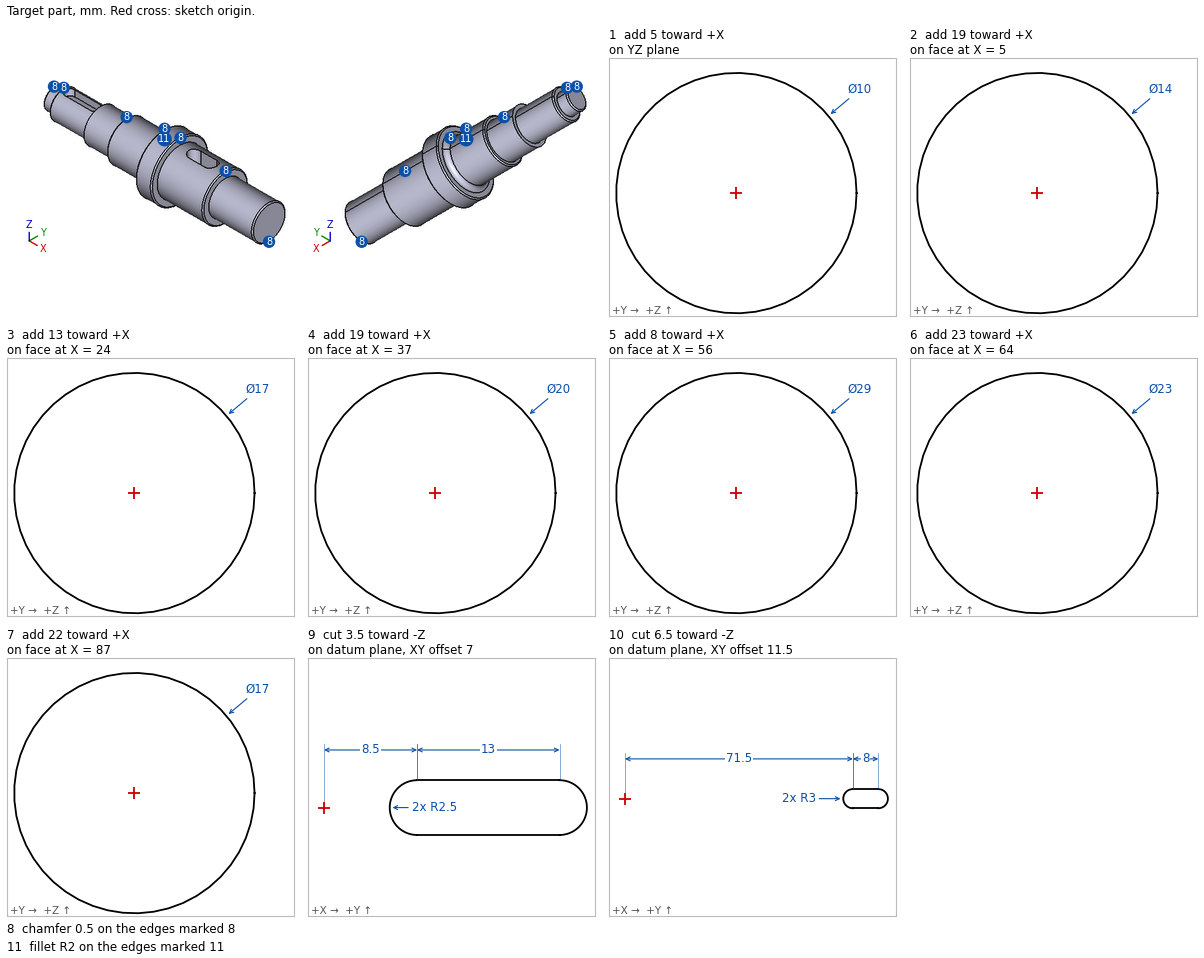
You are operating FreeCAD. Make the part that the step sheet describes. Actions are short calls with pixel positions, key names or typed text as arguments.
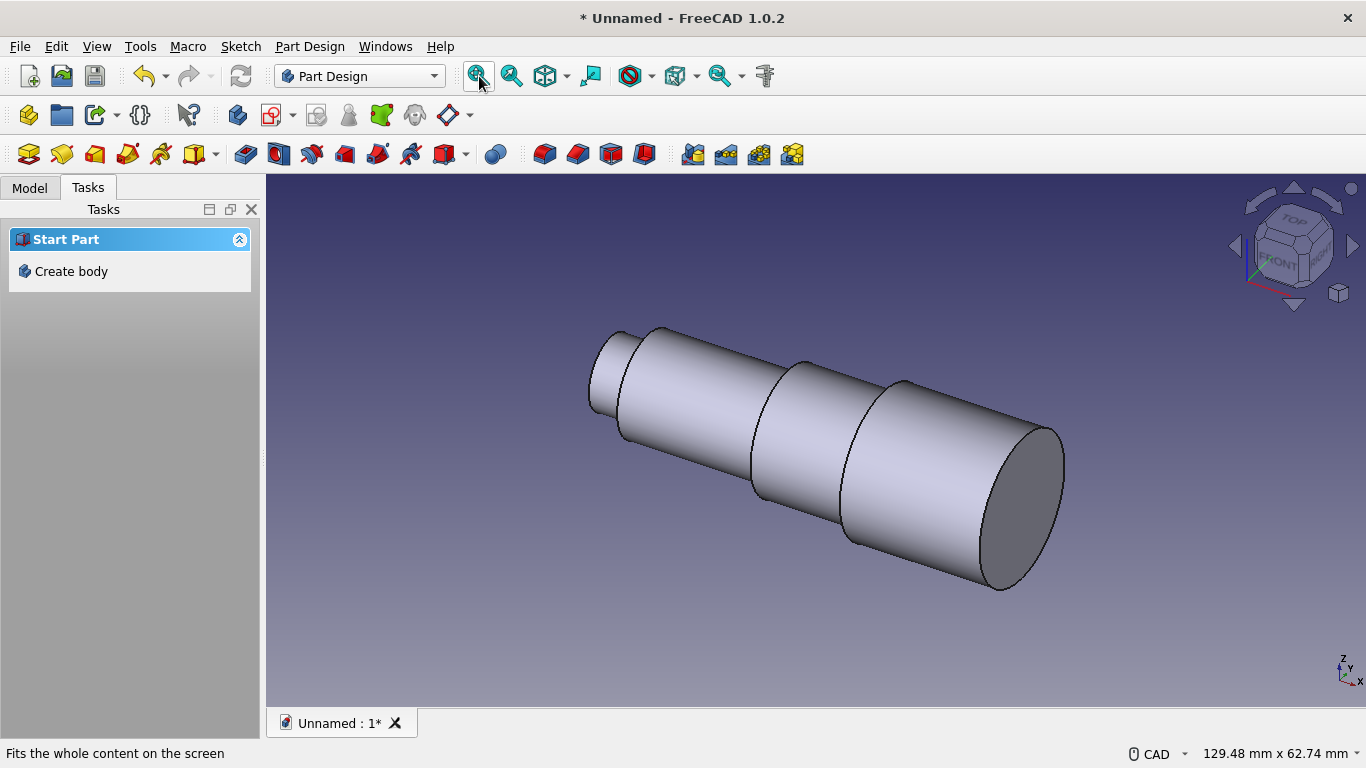
click(1022, 508)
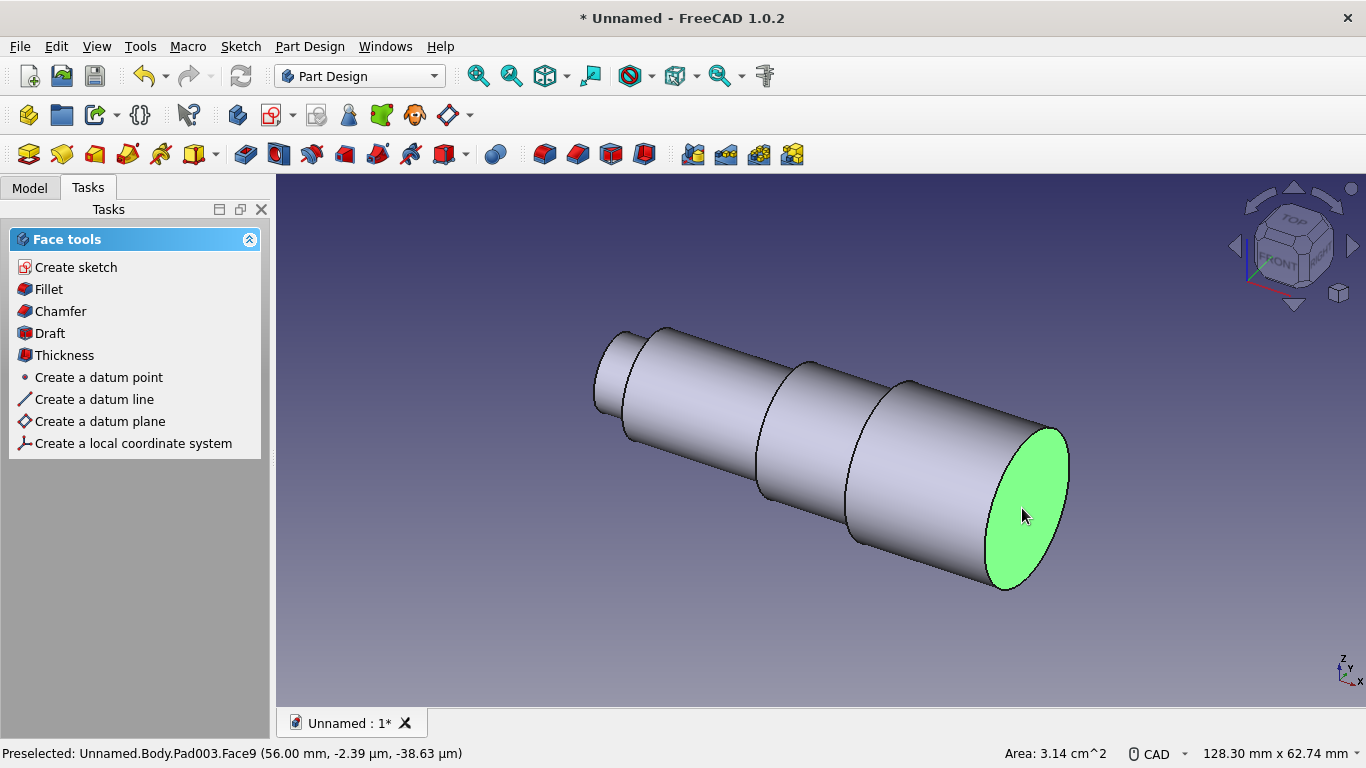
click(270, 116)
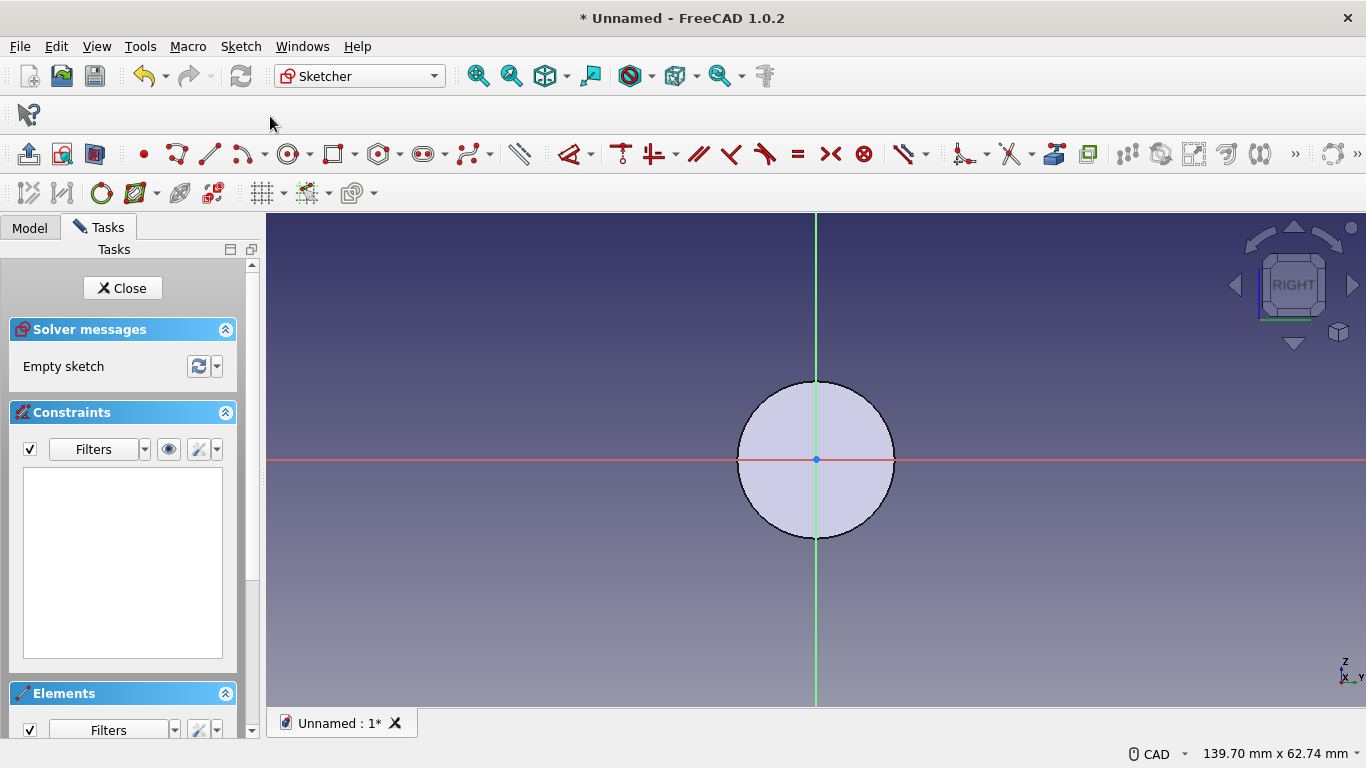
scroll(955, 460, up, 2)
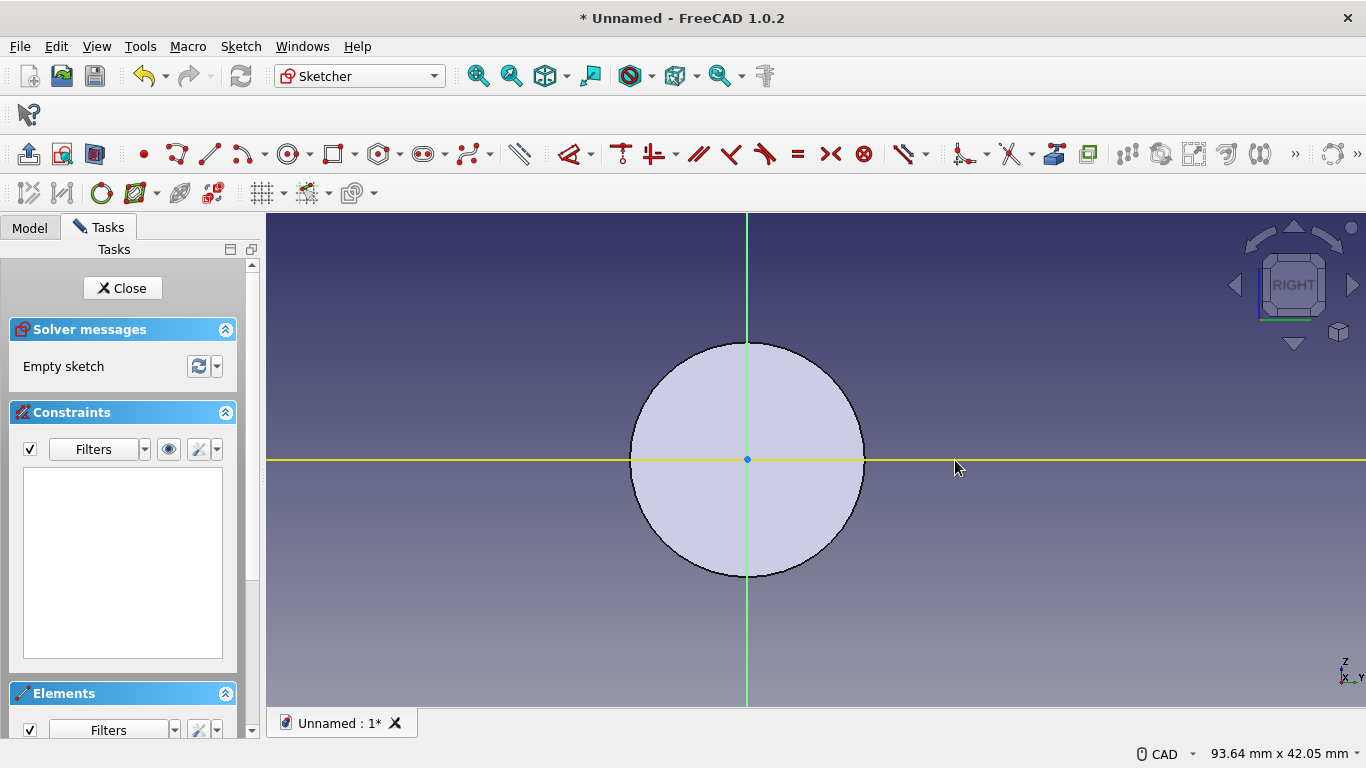
key(g)
key(c)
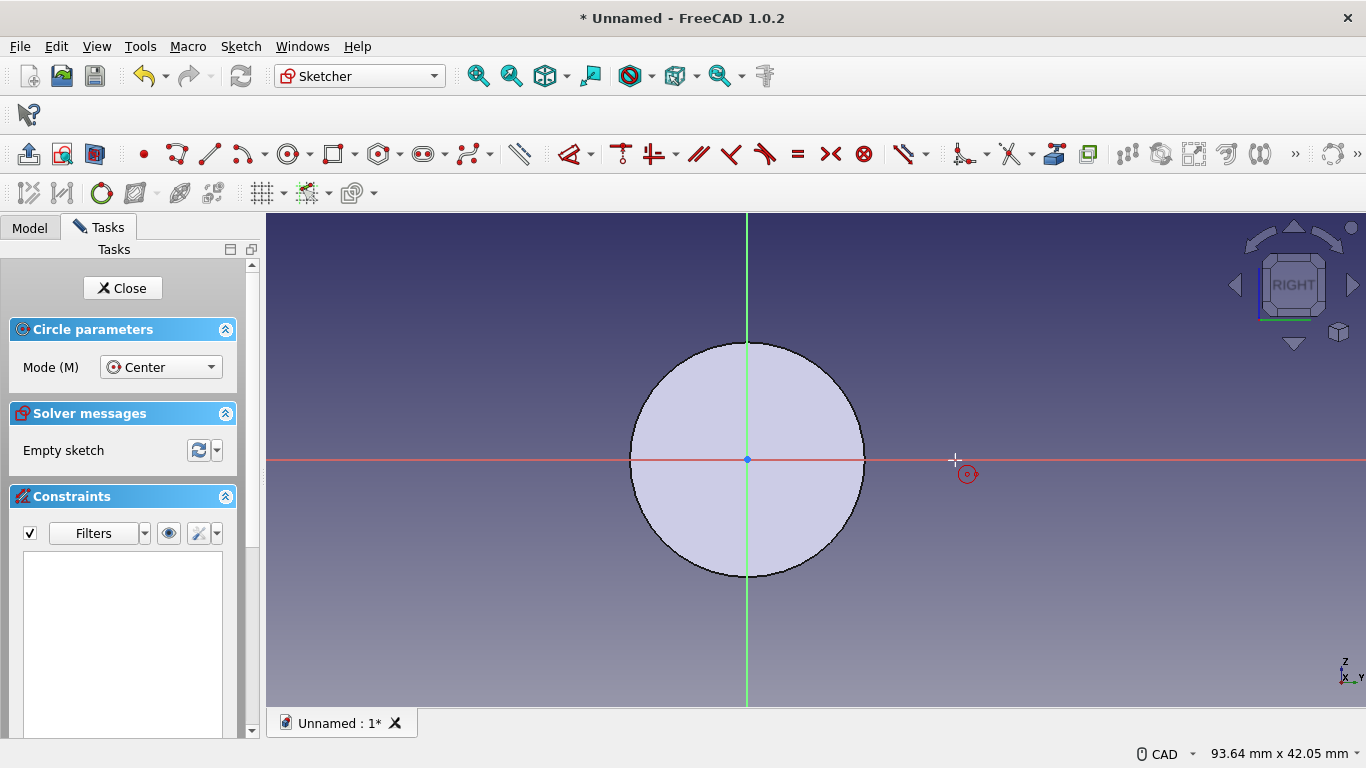
click(747, 460)
move(868, 339)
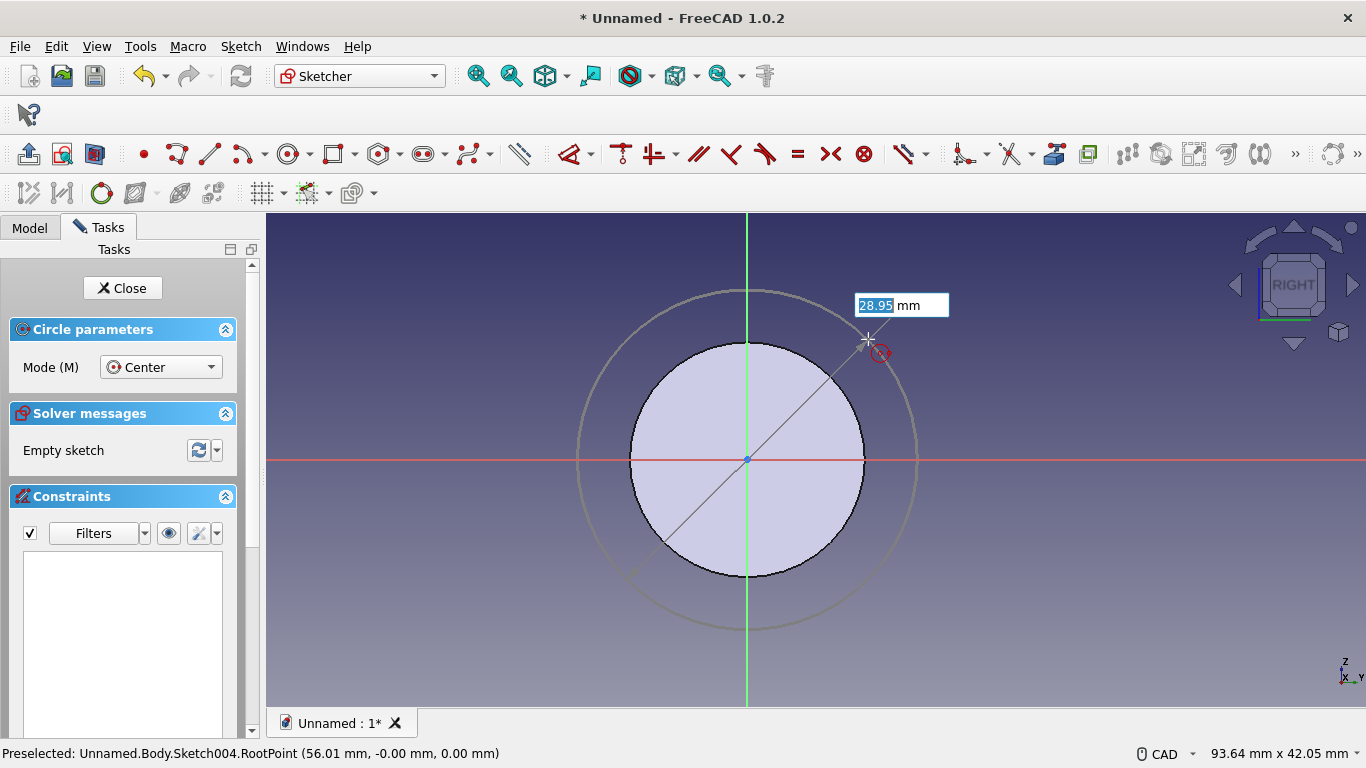
text(29)
key(Return)
key(Escape)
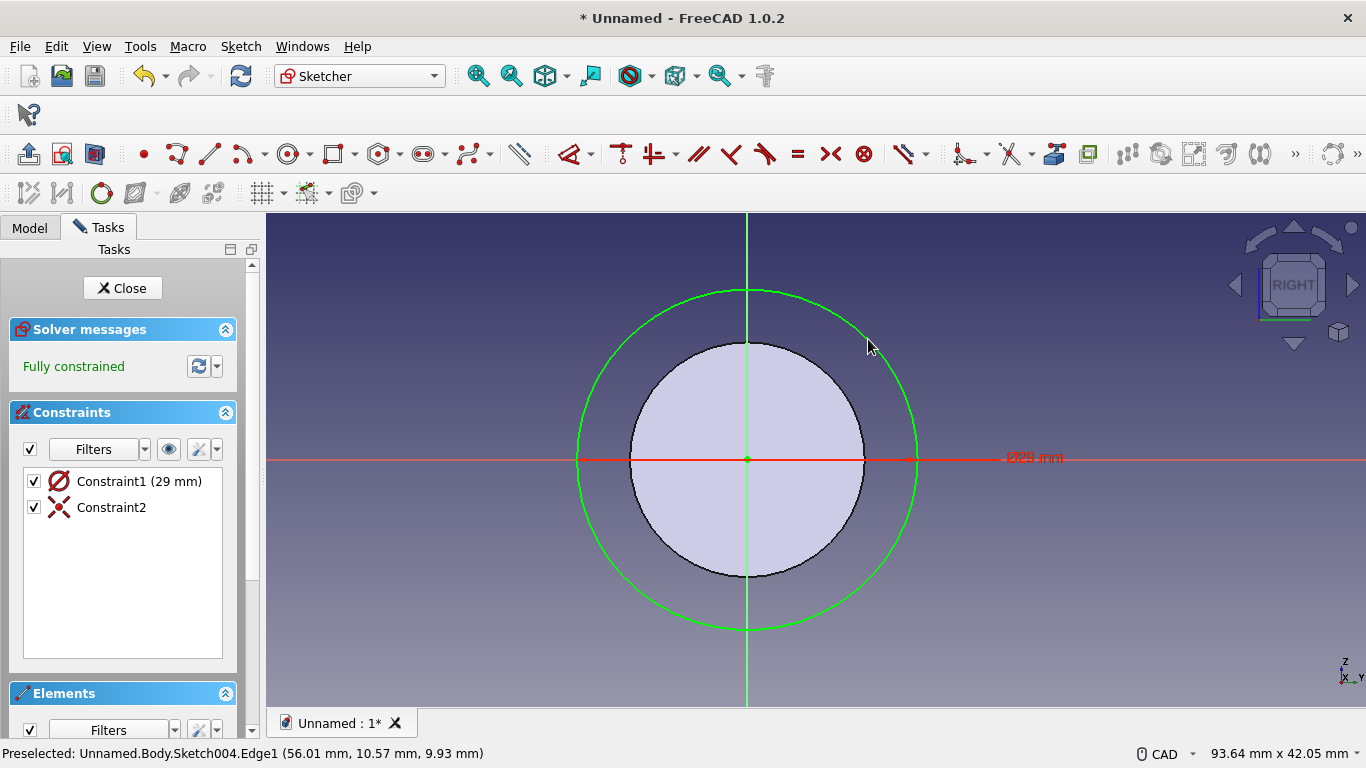
click(123, 288)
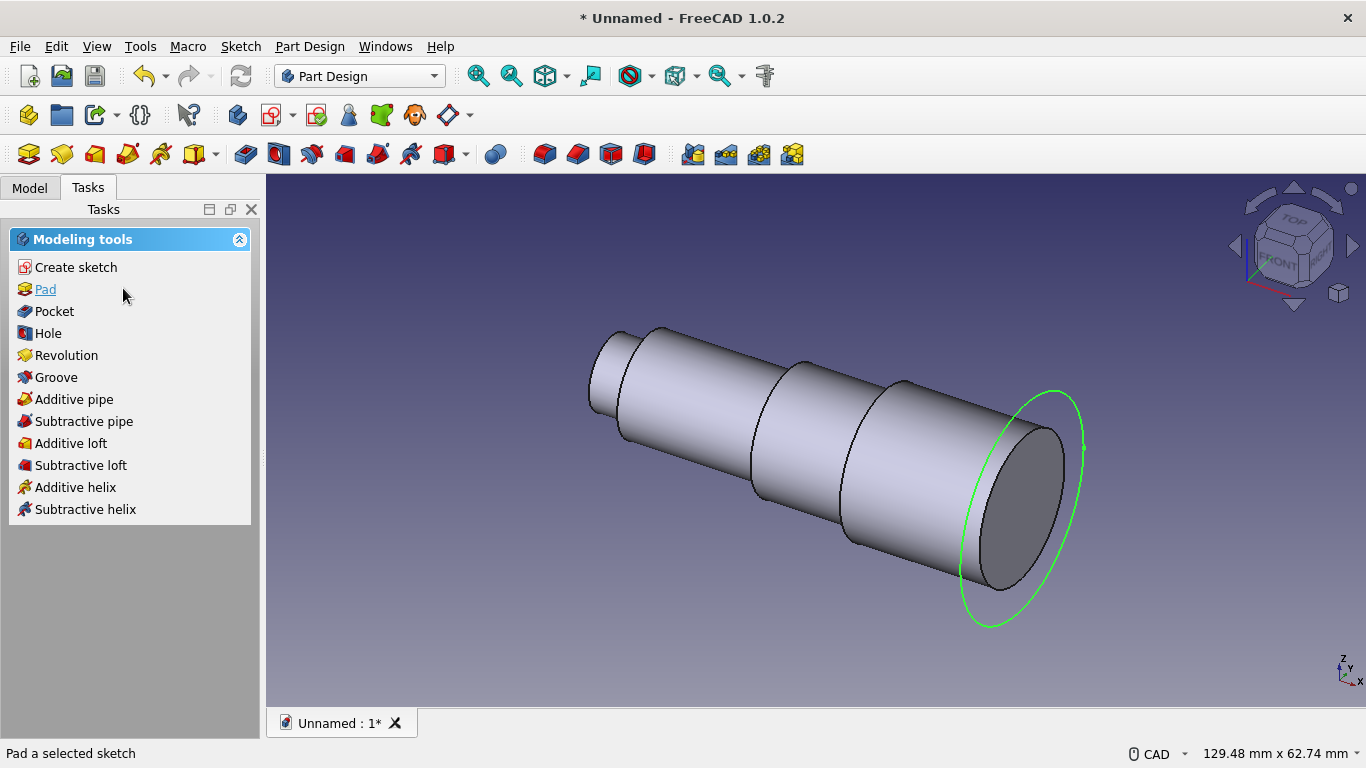
click(29, 154)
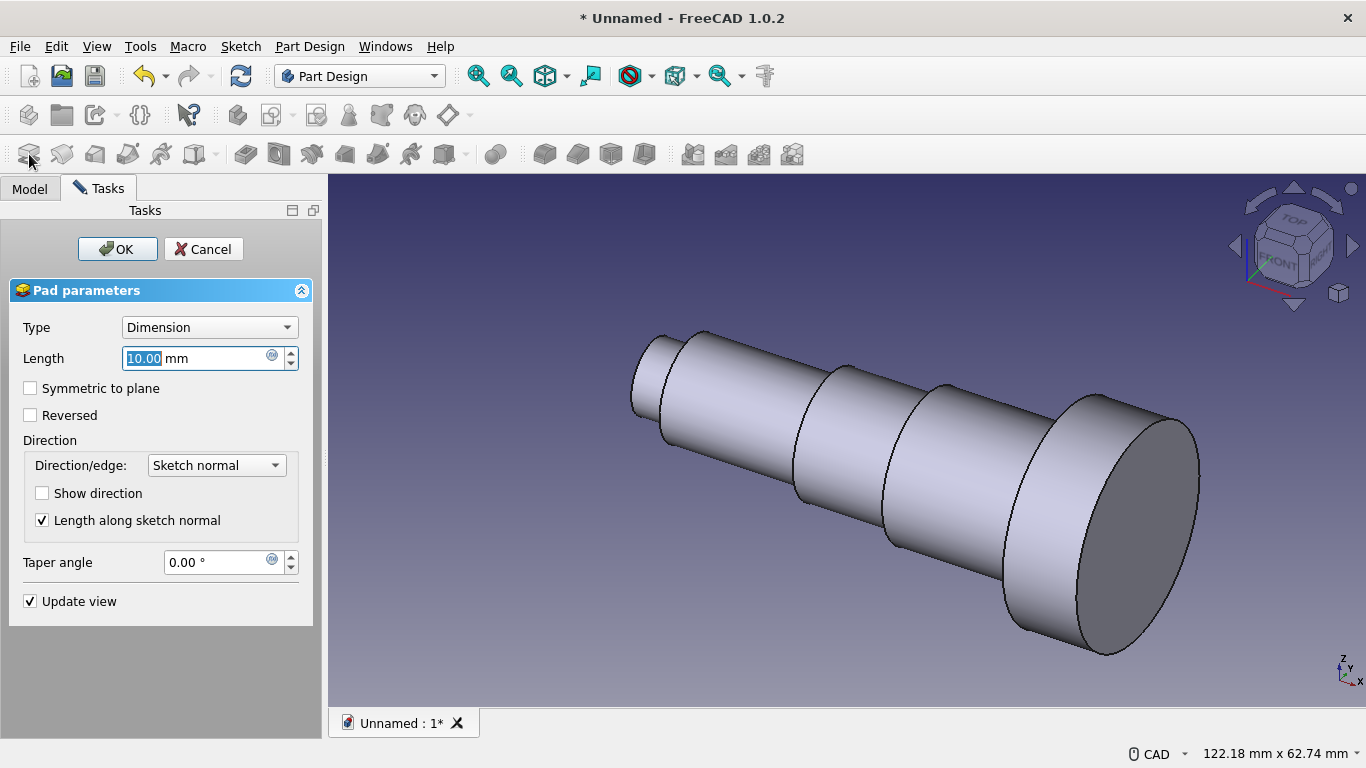
text(8)
key(Tab)